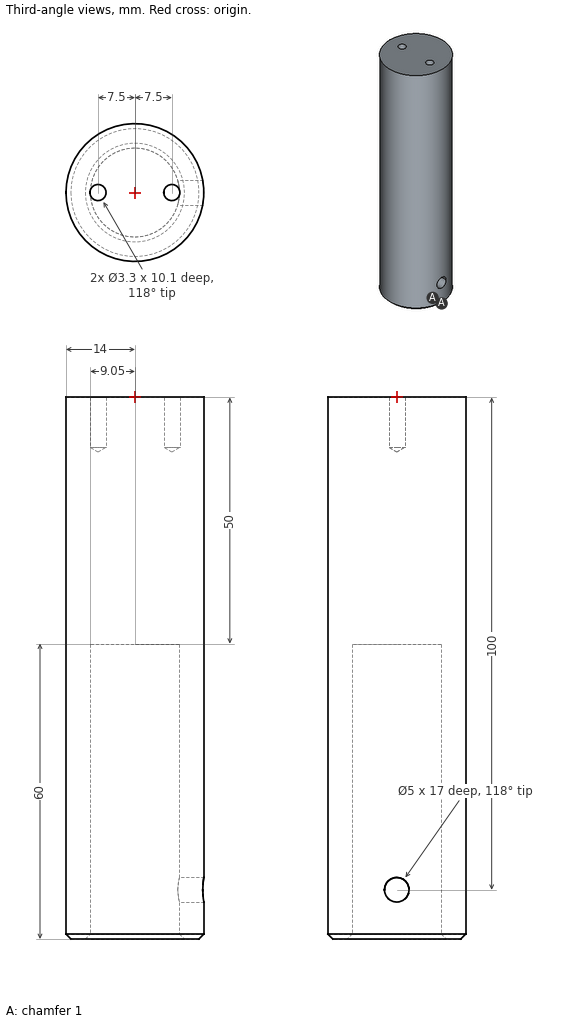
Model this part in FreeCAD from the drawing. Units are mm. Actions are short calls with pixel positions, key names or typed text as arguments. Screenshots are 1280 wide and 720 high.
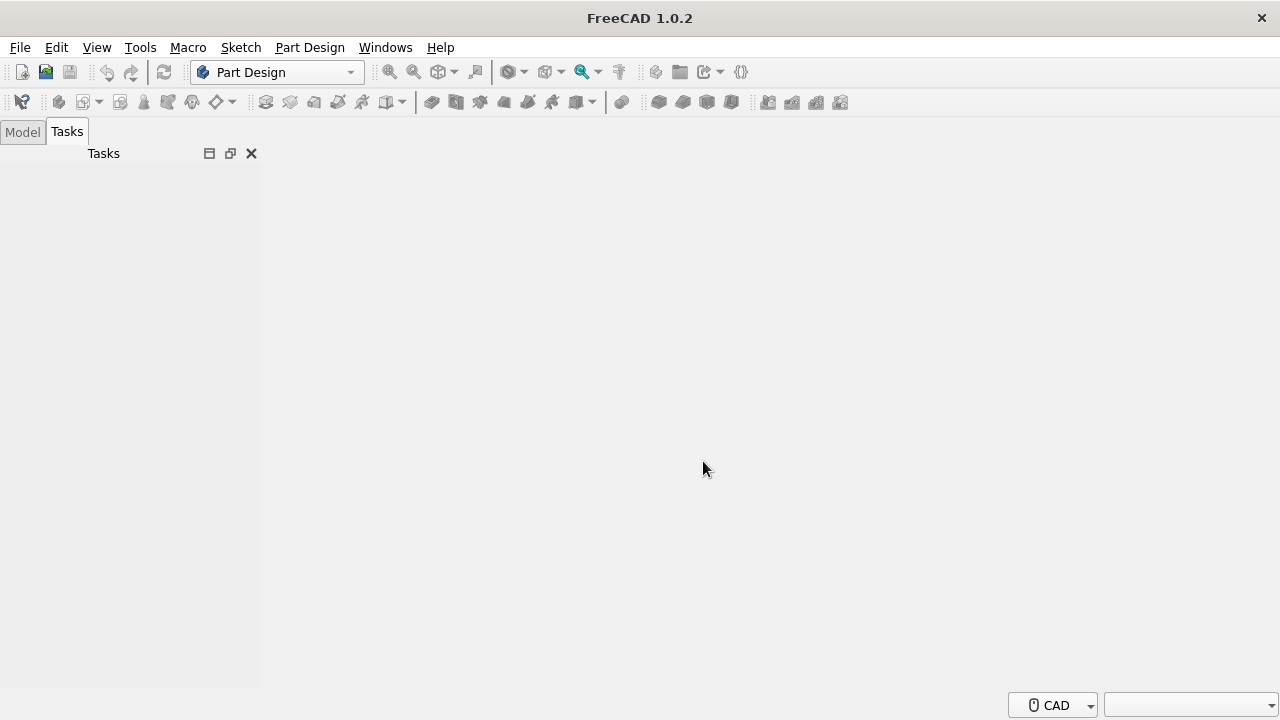
click(22, 72)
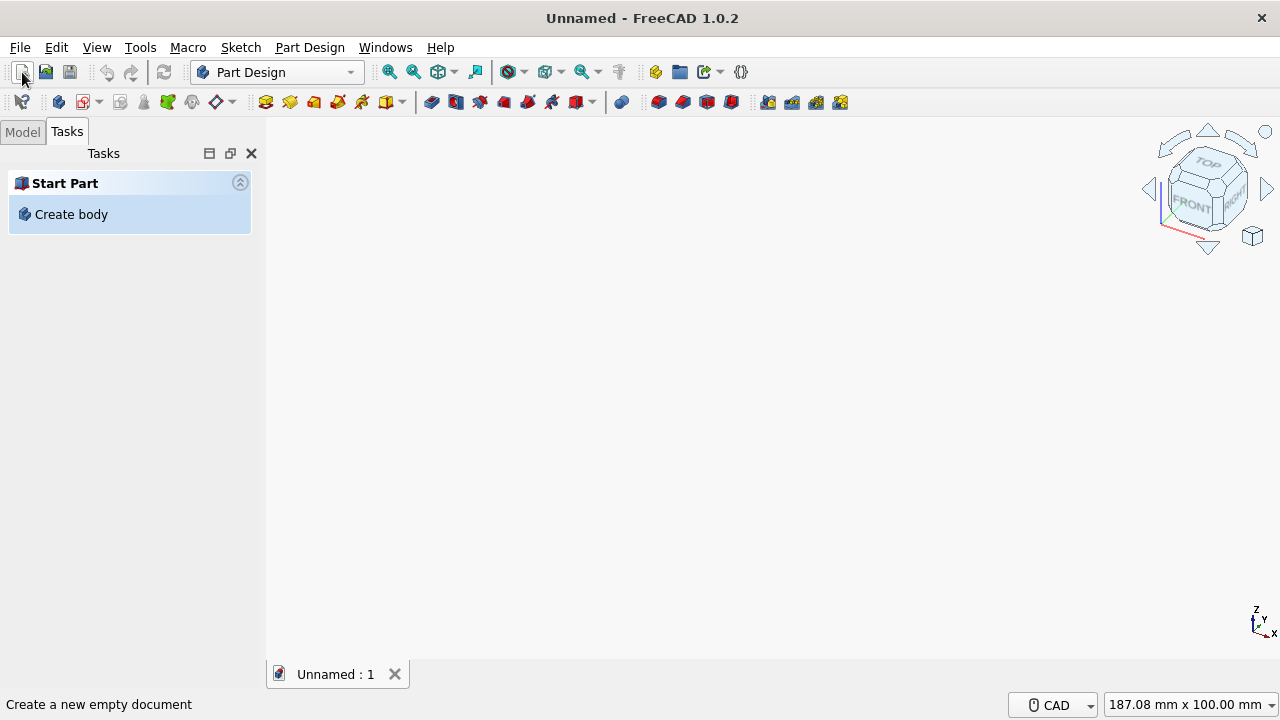
click(84, 102)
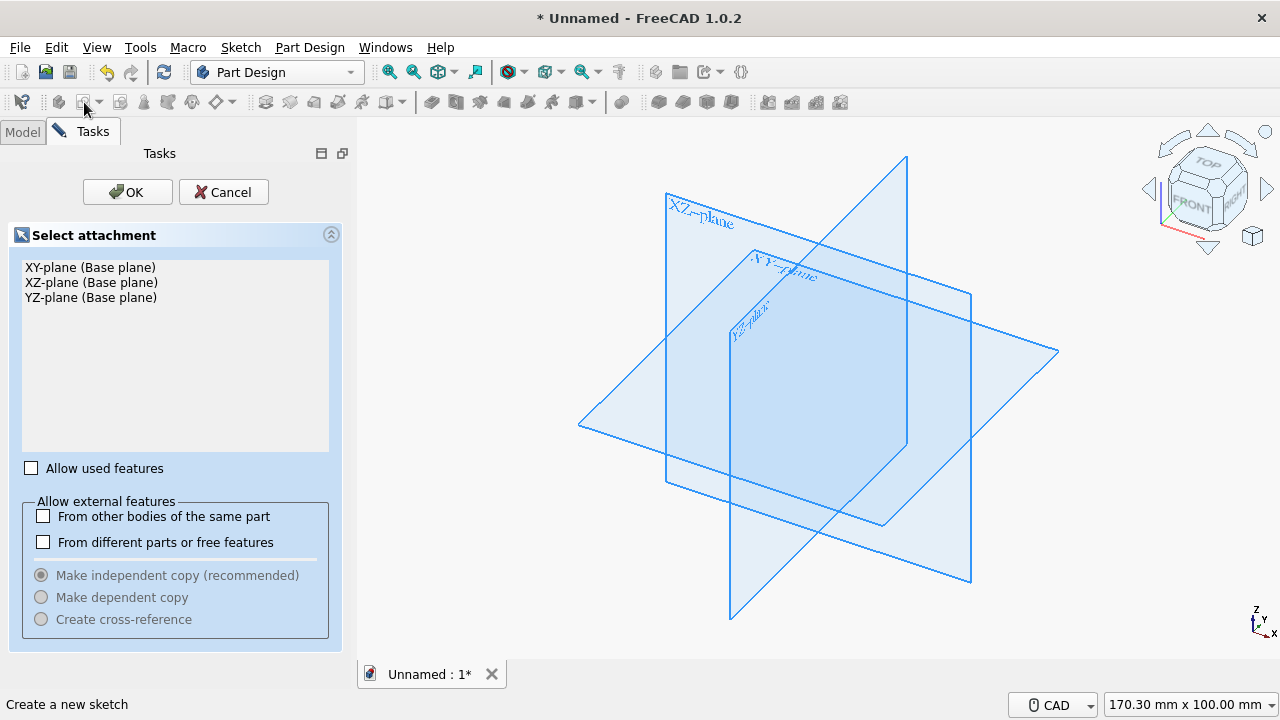
click(82, 282)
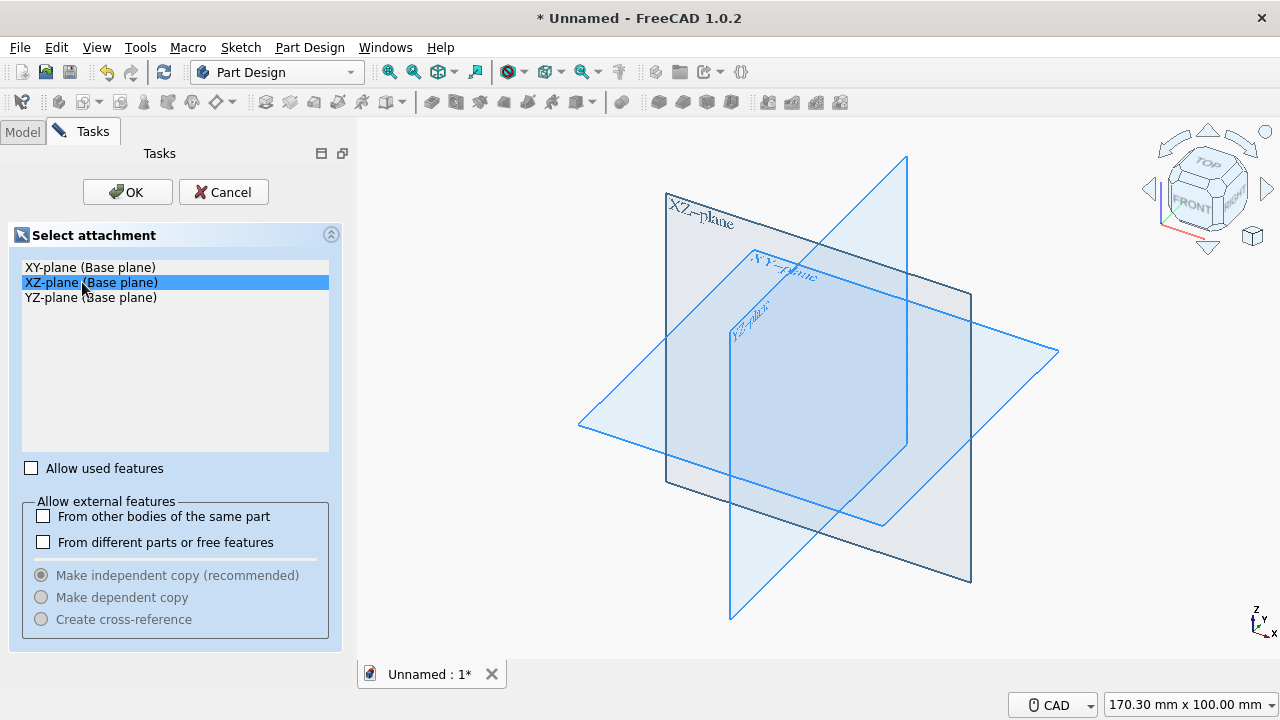
click(128, 192)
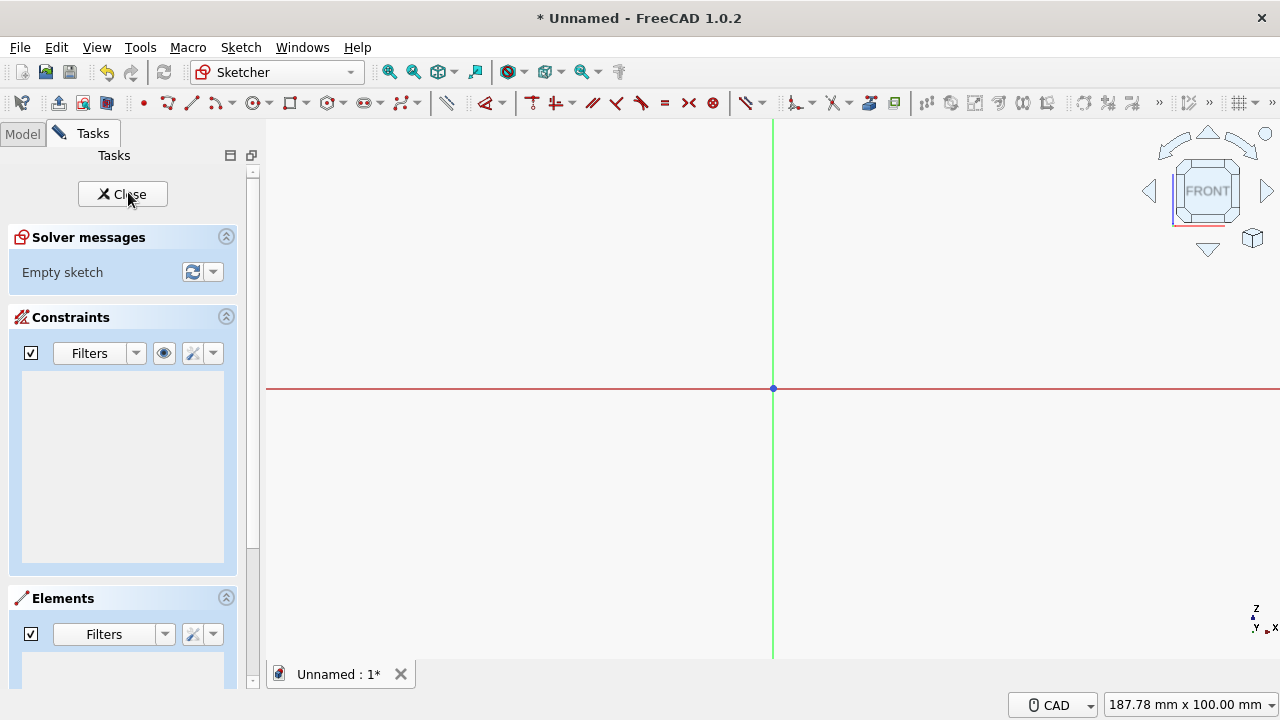
scroll(667, 147, down, 3)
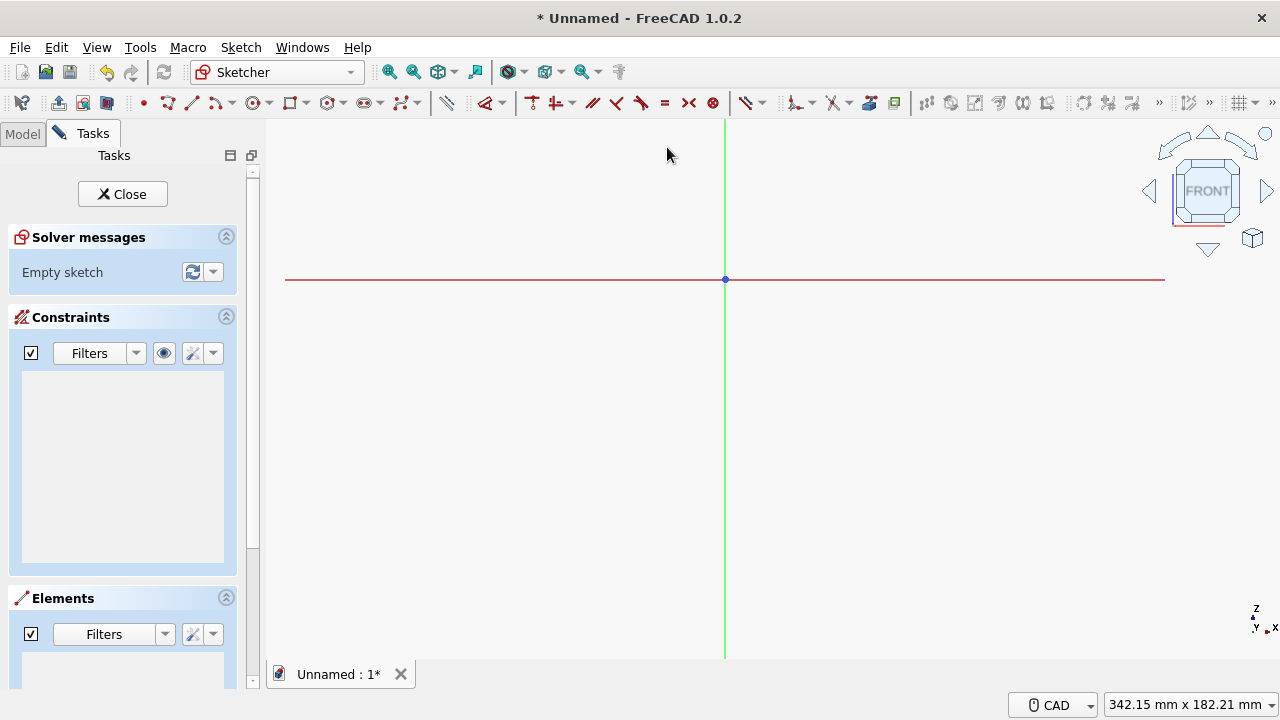
click(168, 104)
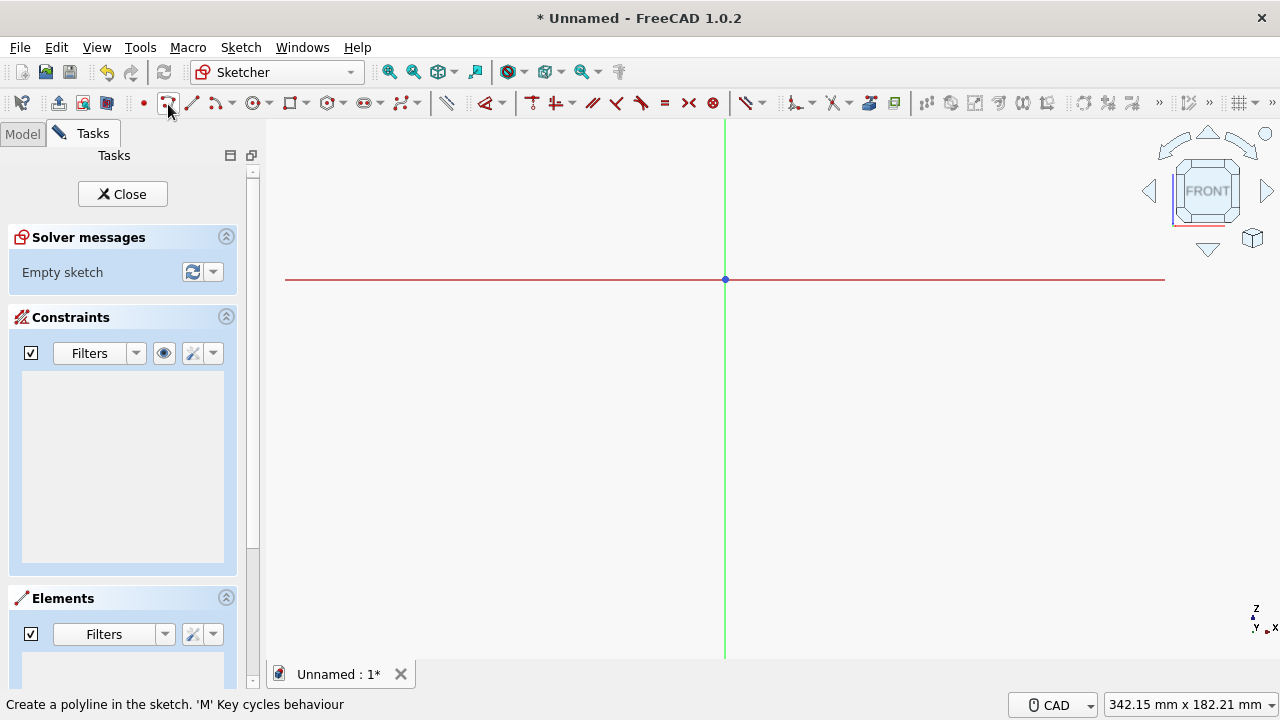
click(725, 280)
click(716, 428)
click(699, 428)
click(699, 606)
click(684, 606)
click(684, 289)
click(725, 280)
key(Escape)
key(Escape)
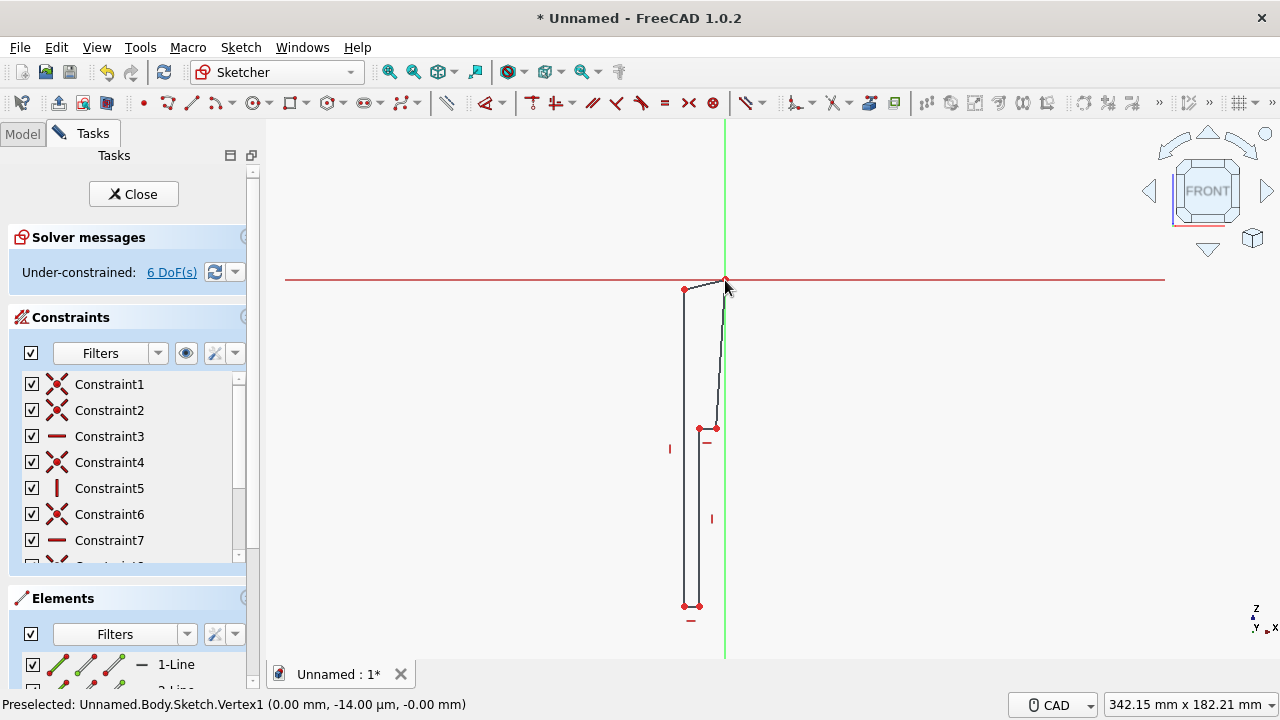
click(723, 325)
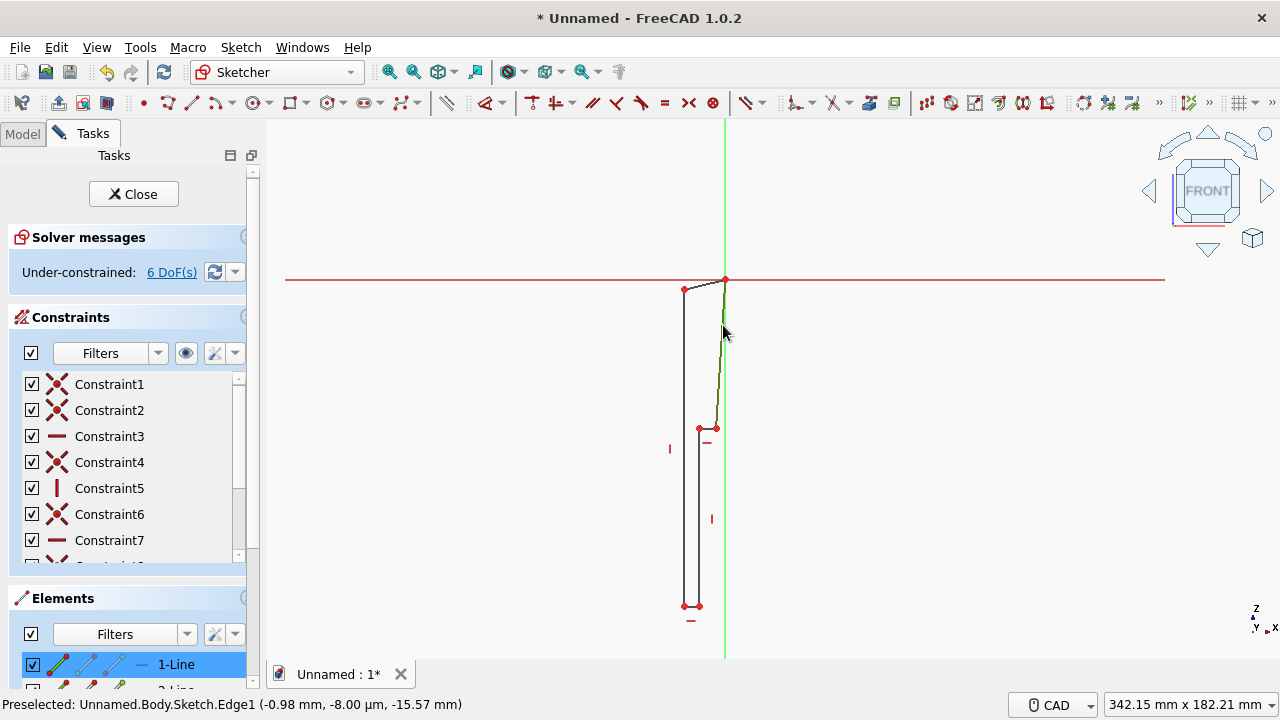
click(574, 104)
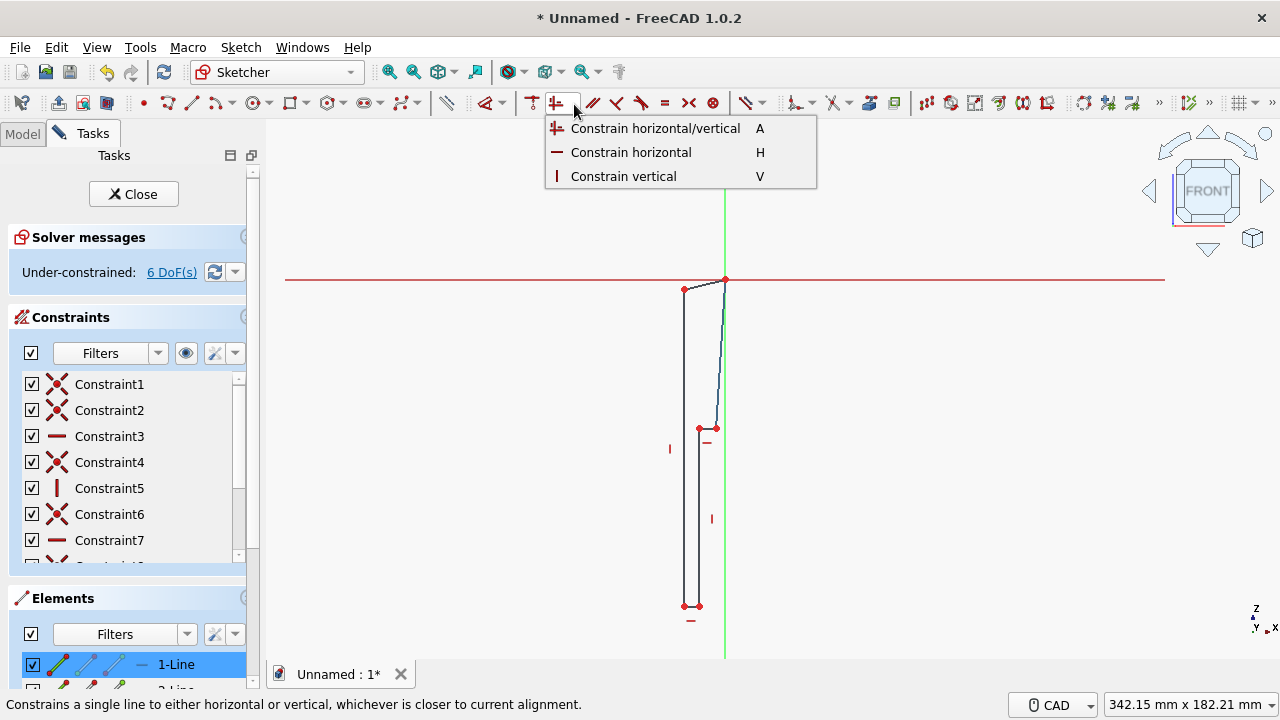
click(681, 176)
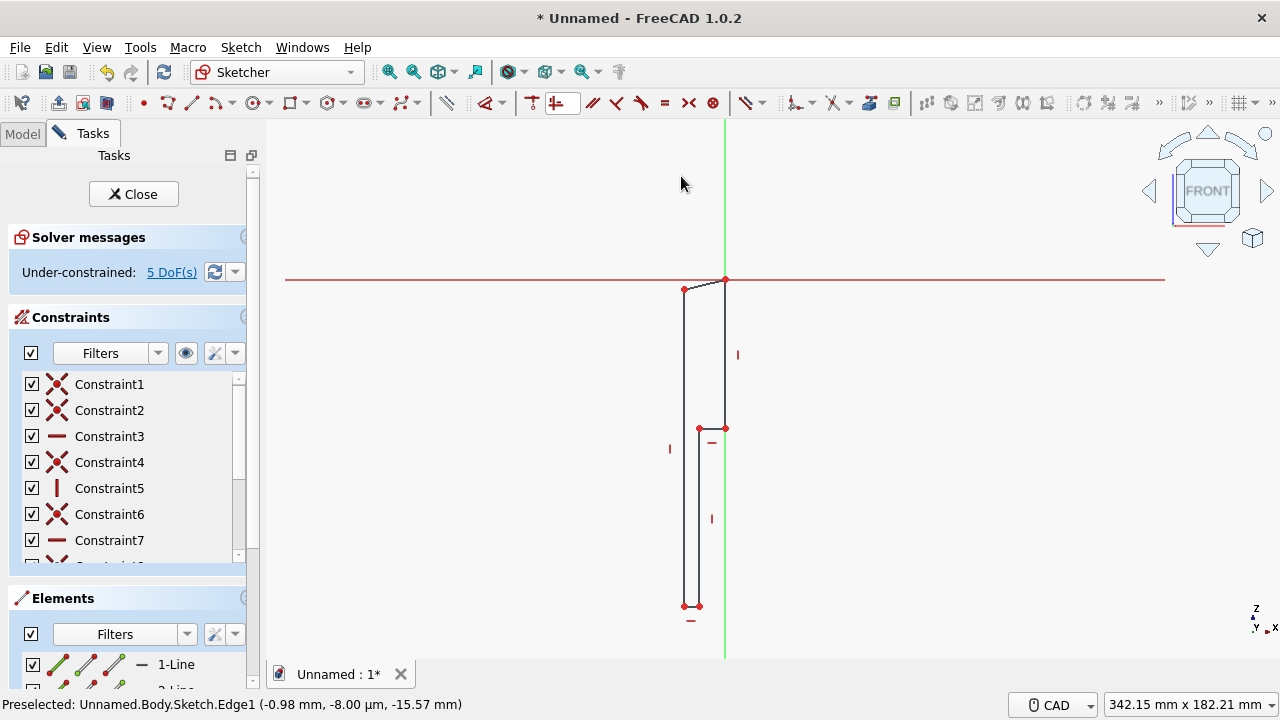
click(713, 283)